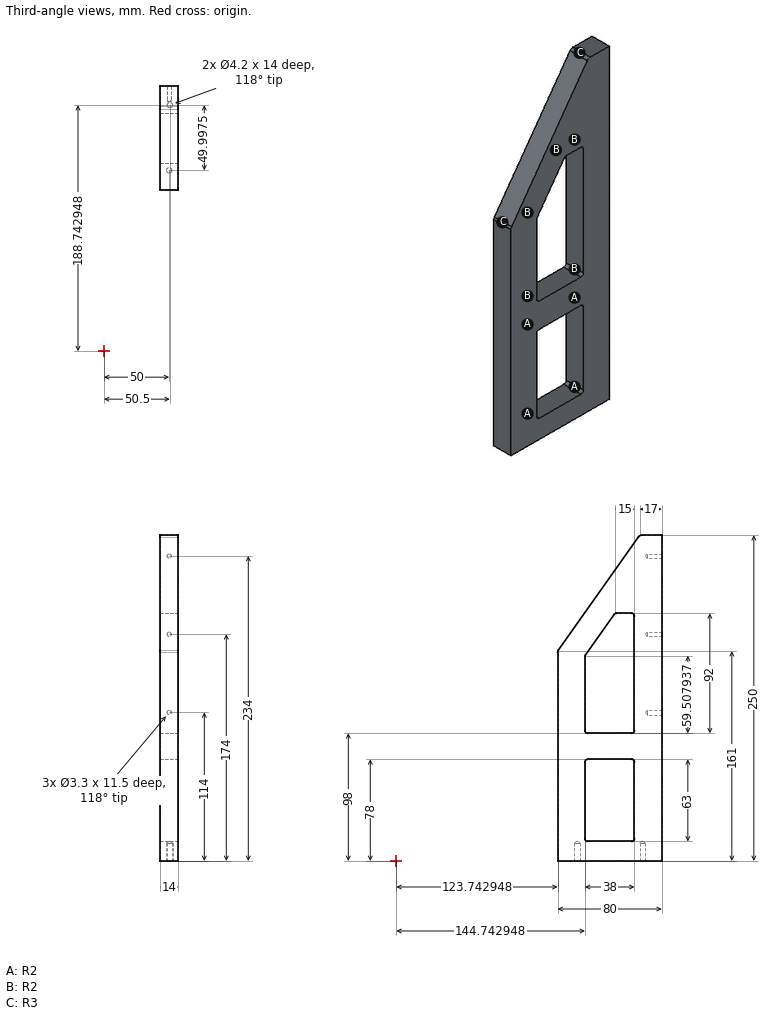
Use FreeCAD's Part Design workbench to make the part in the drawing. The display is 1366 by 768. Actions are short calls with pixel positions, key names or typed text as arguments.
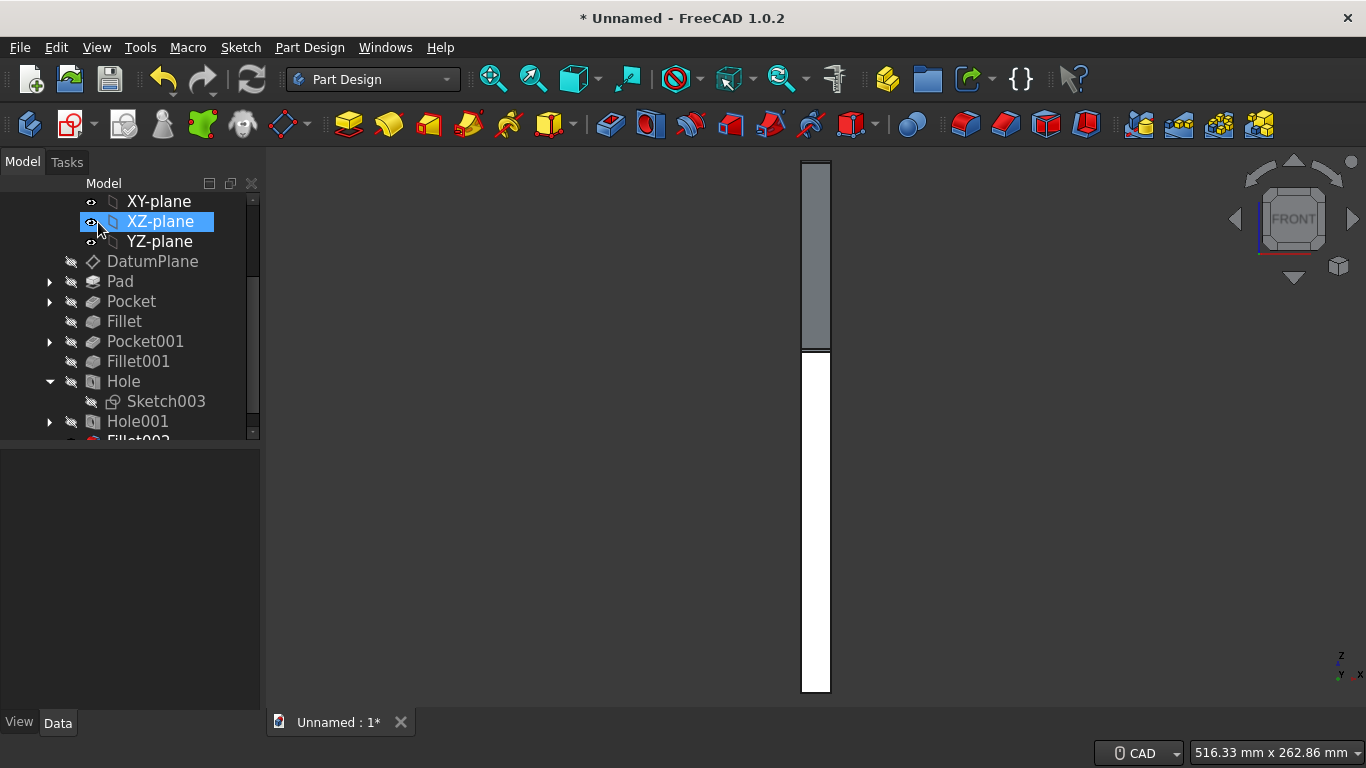
key(0)